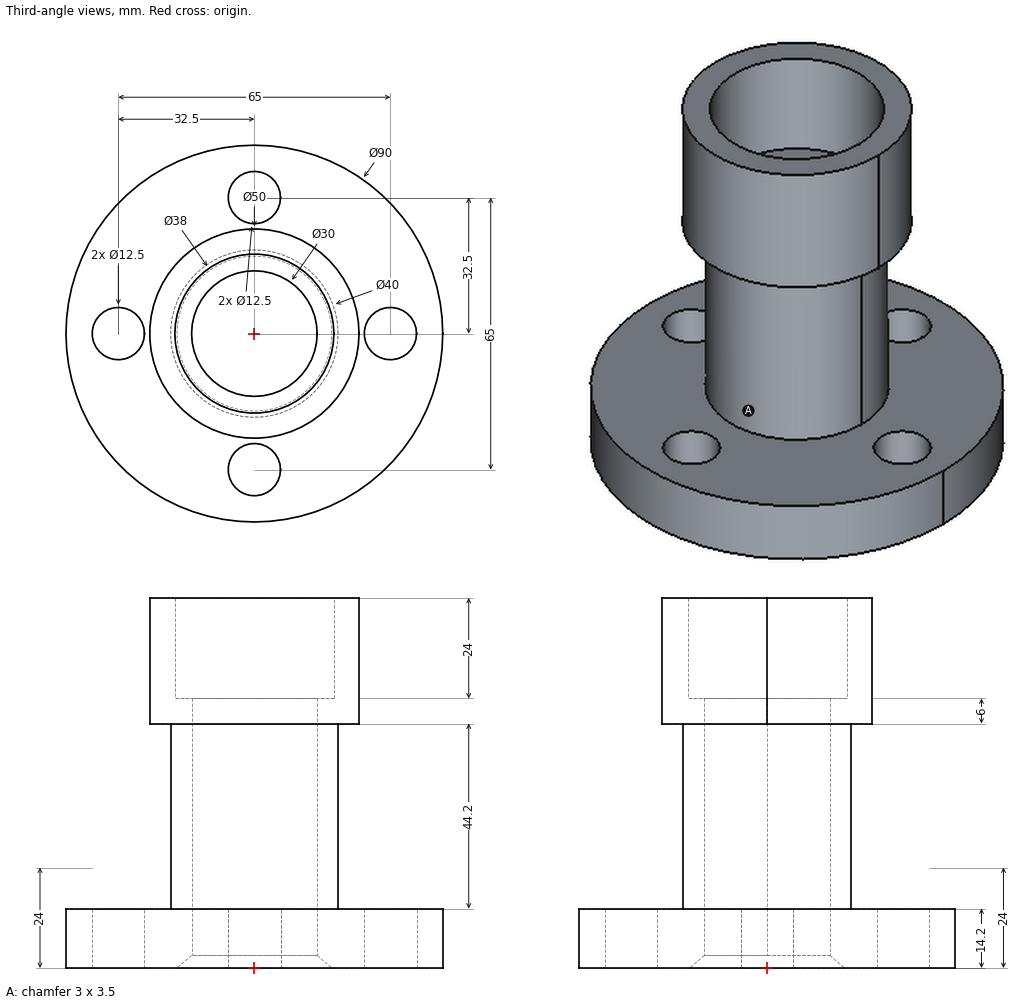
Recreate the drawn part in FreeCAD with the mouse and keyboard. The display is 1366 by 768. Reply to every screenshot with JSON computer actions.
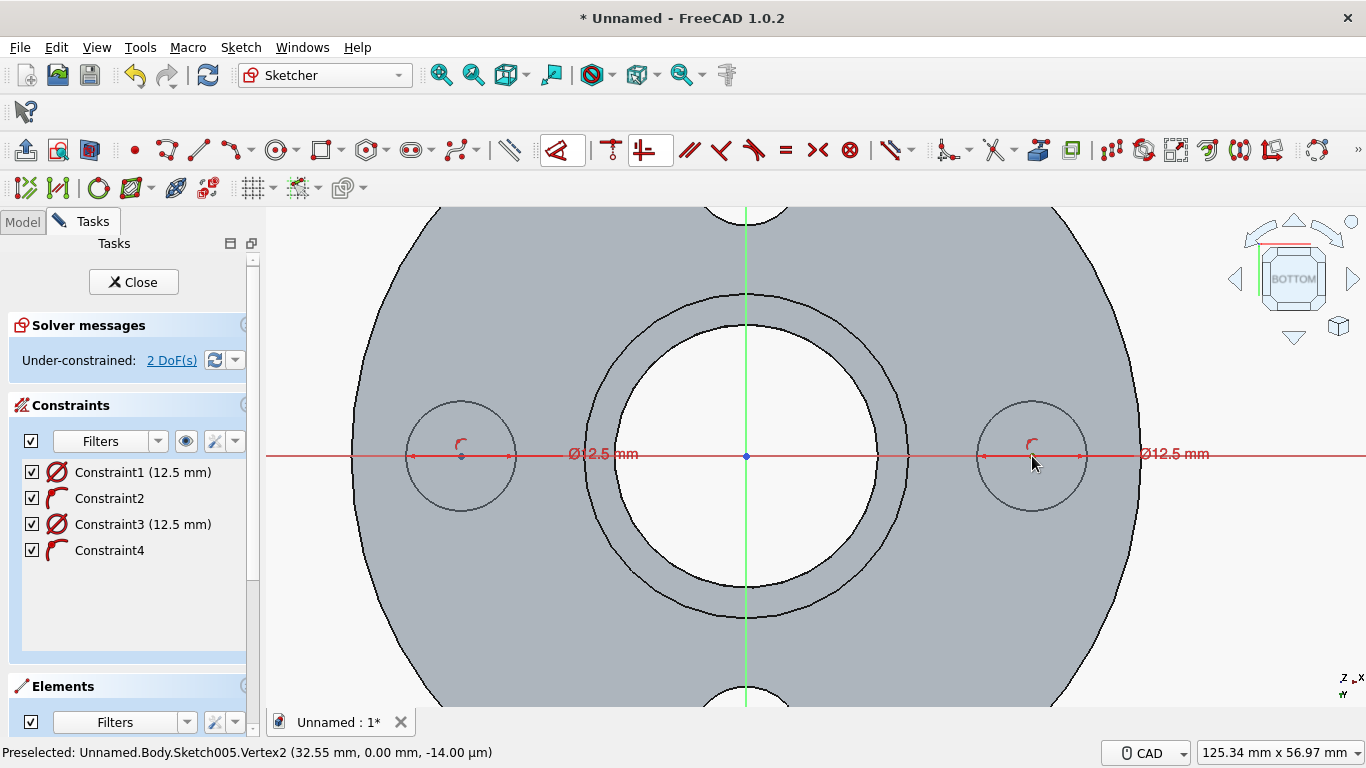
{"action": "left_click", "coordinate": [580, 150]}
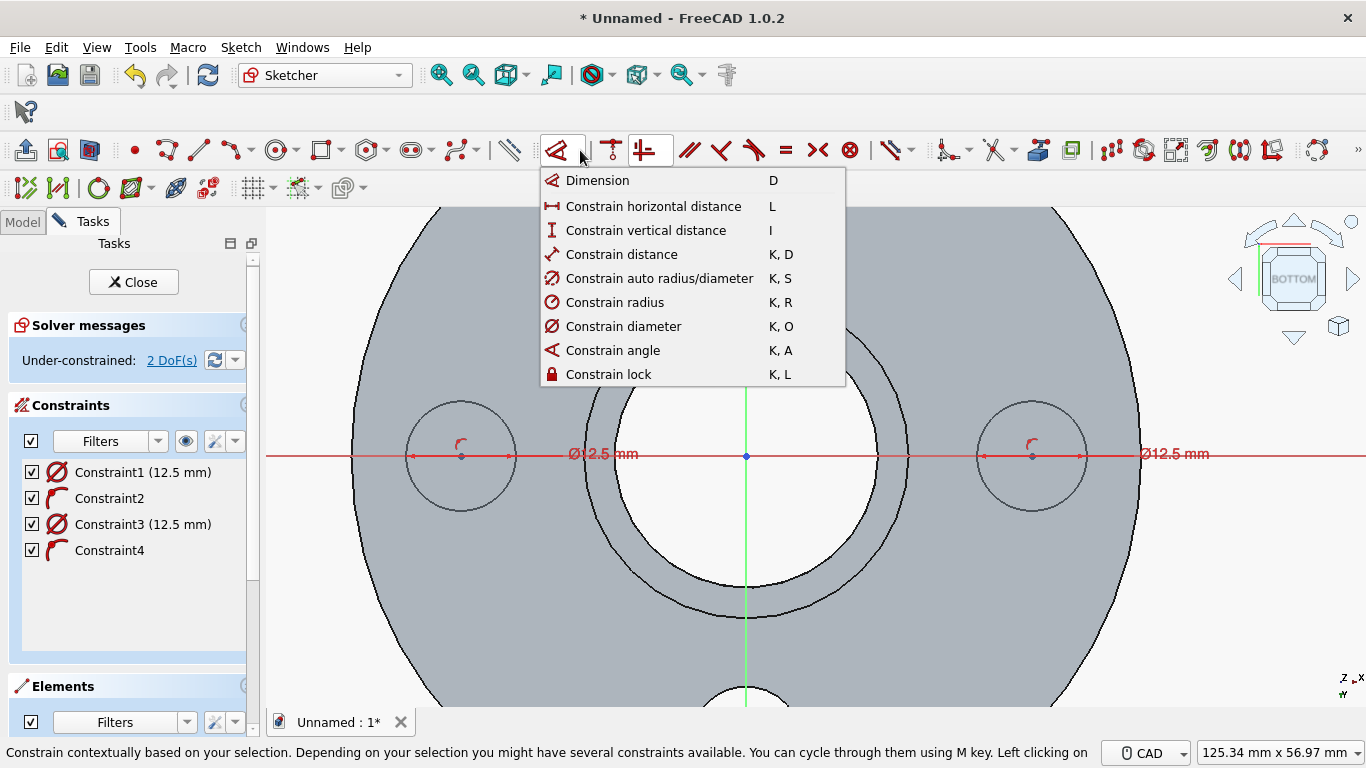
{"action": "left_click", "coordinate": [693, 206]}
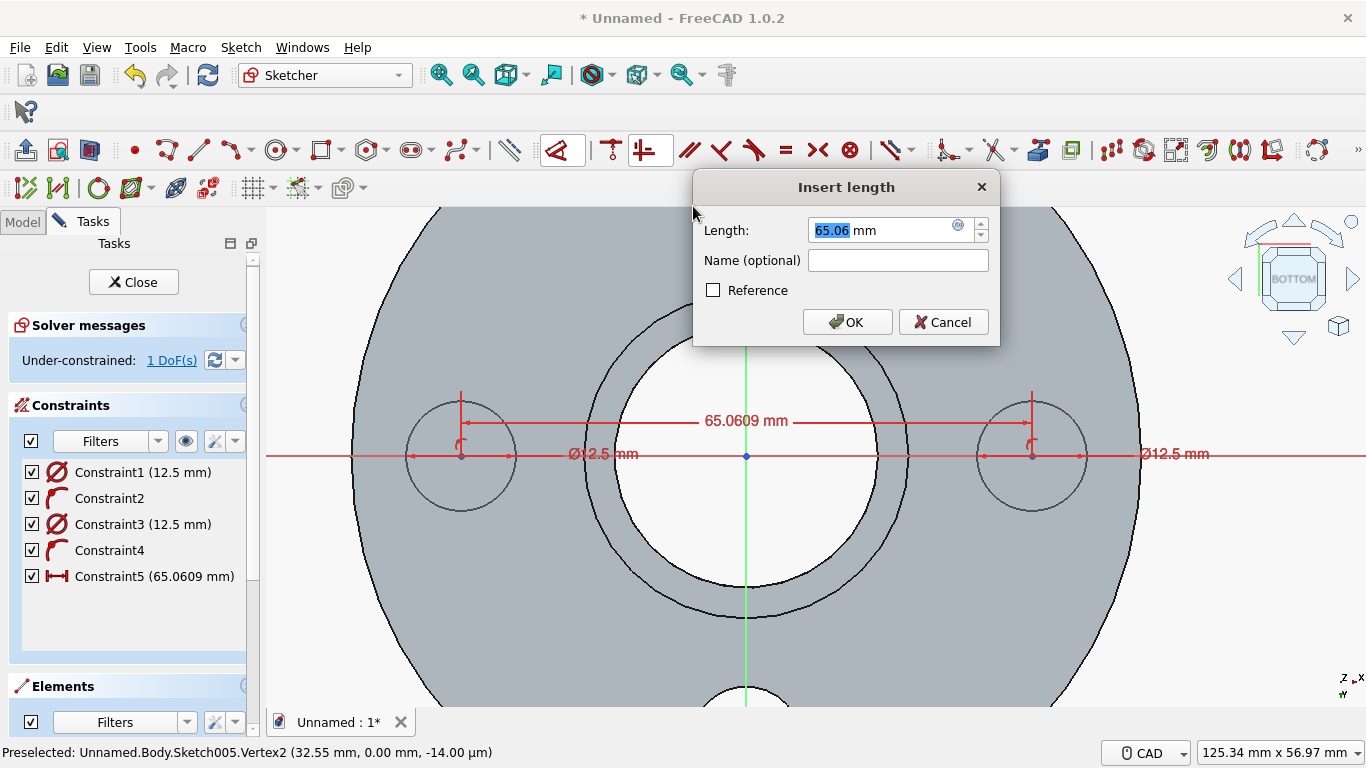
{"action": "type", "text": "65"}
{"action": "key", "text": "Return"}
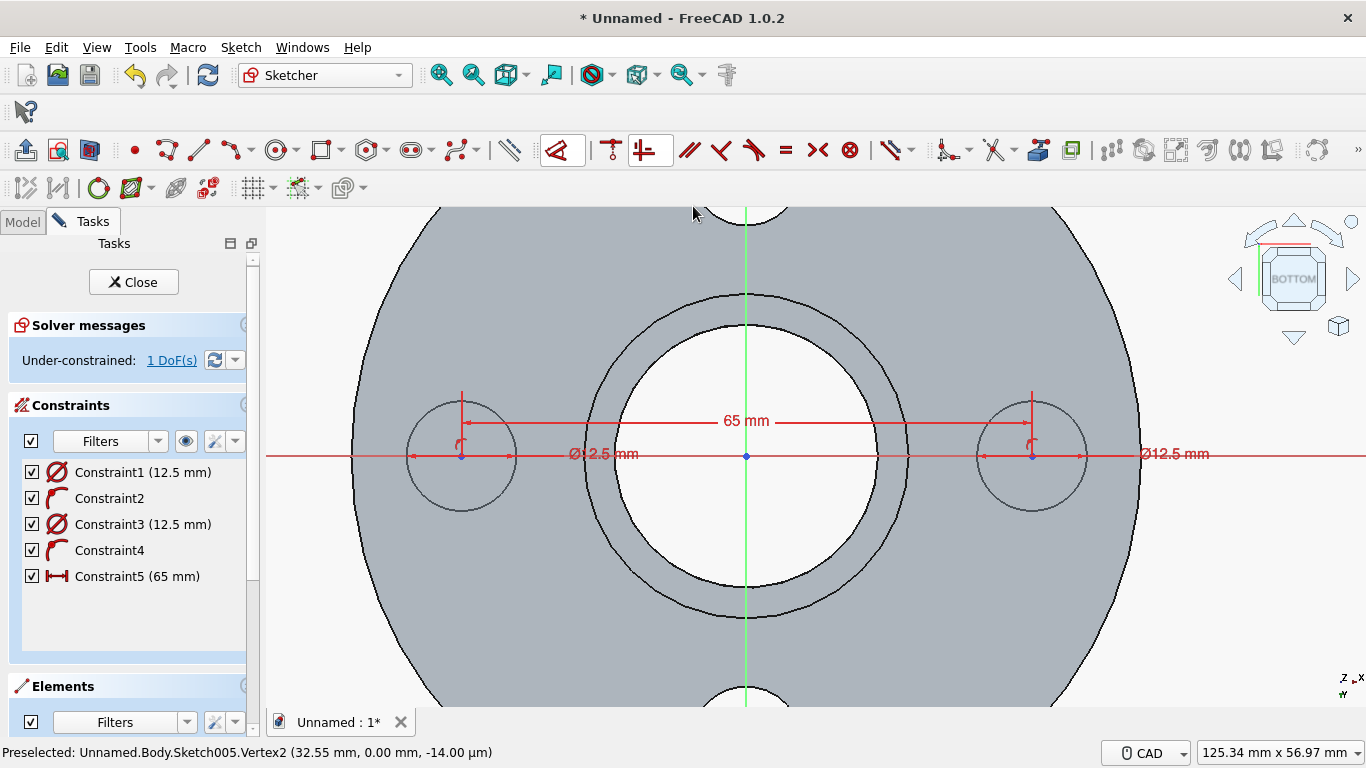
{"action": "left_click", "coordinate": [462, 456]}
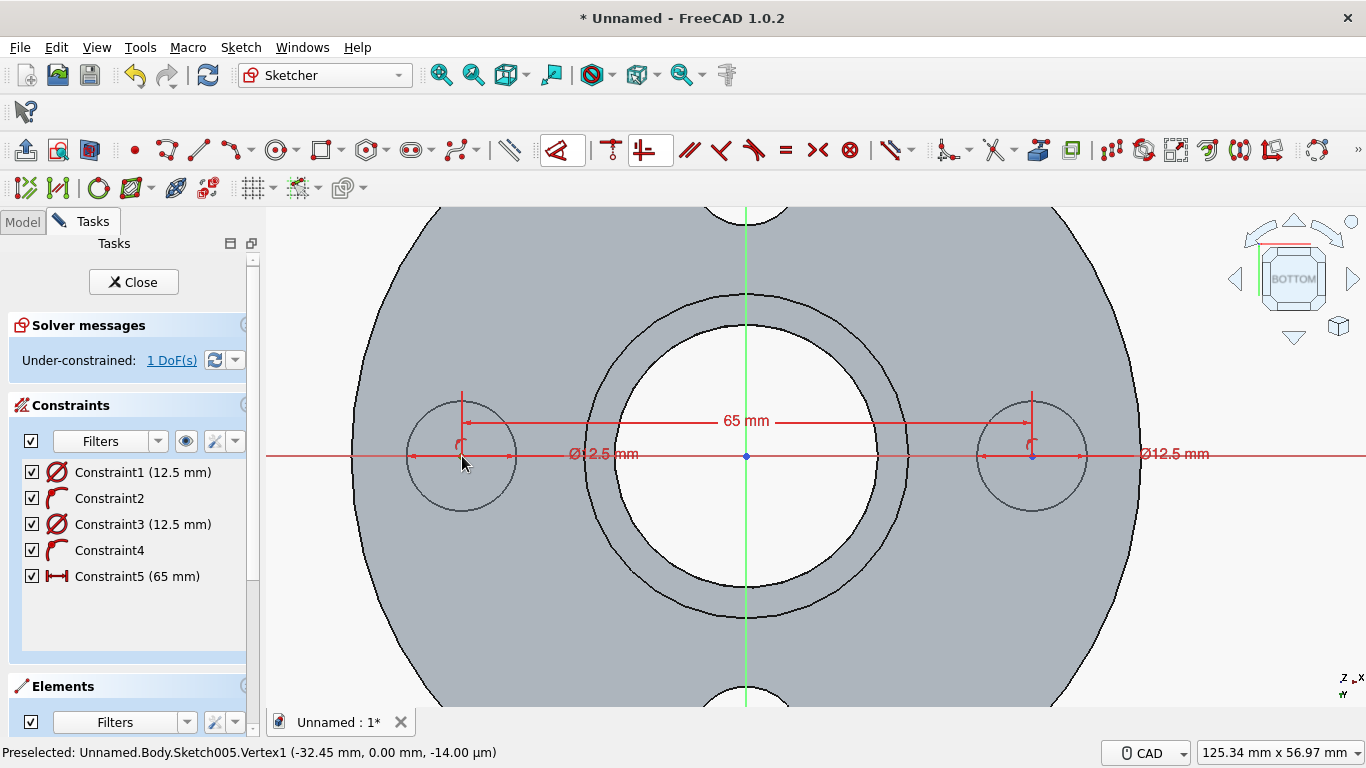
{"action": "left_click", "coordinate": [580, 150]}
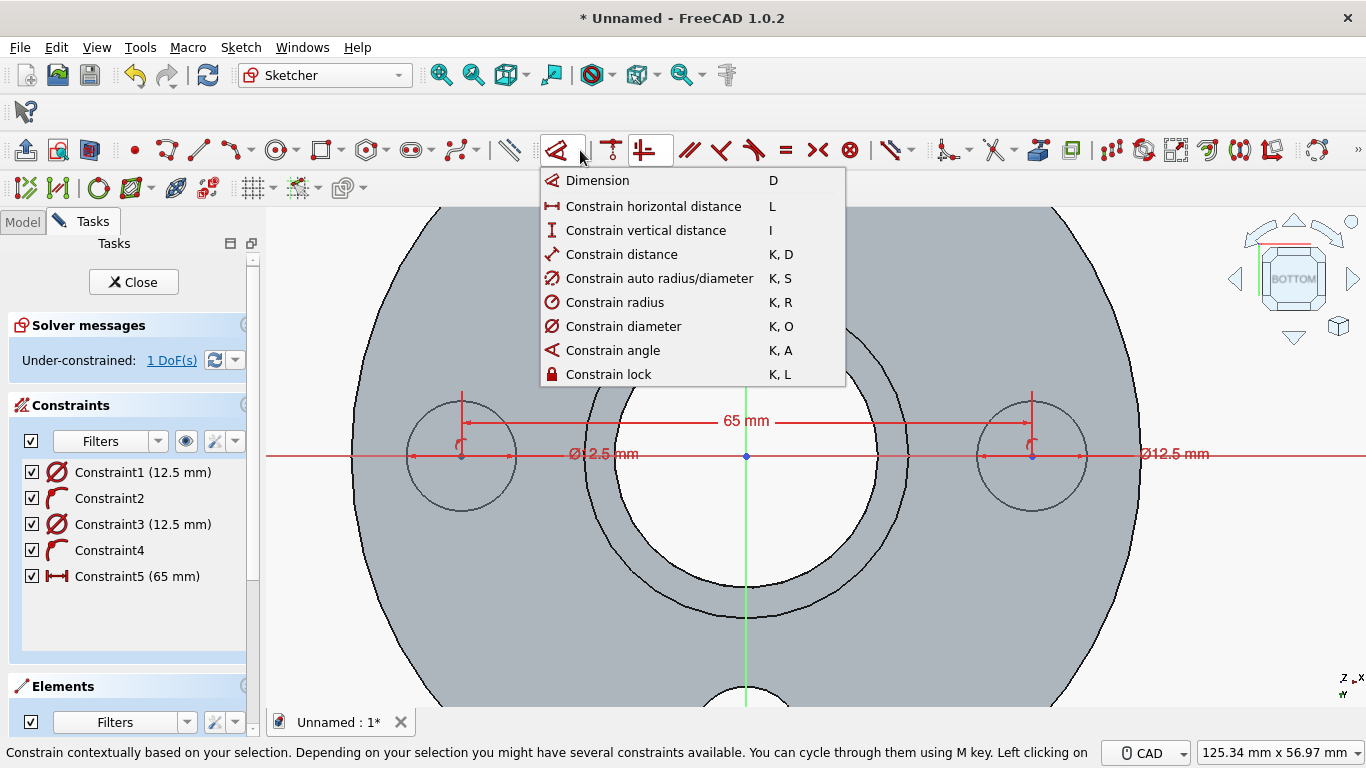
{"action": "left_click", "coordinate": [693, 206]}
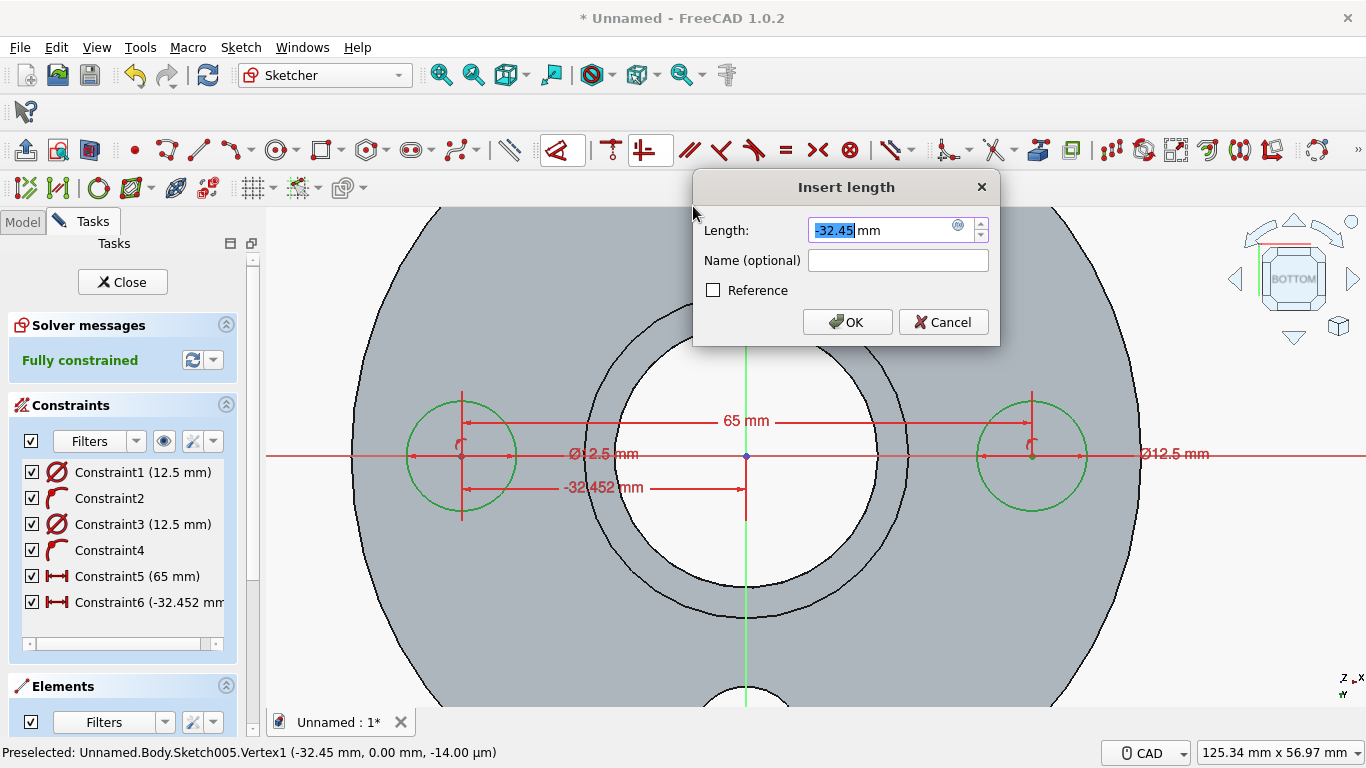
{"action": "type", "text": "-32.5"}
{"action": "key", "text": "Return"}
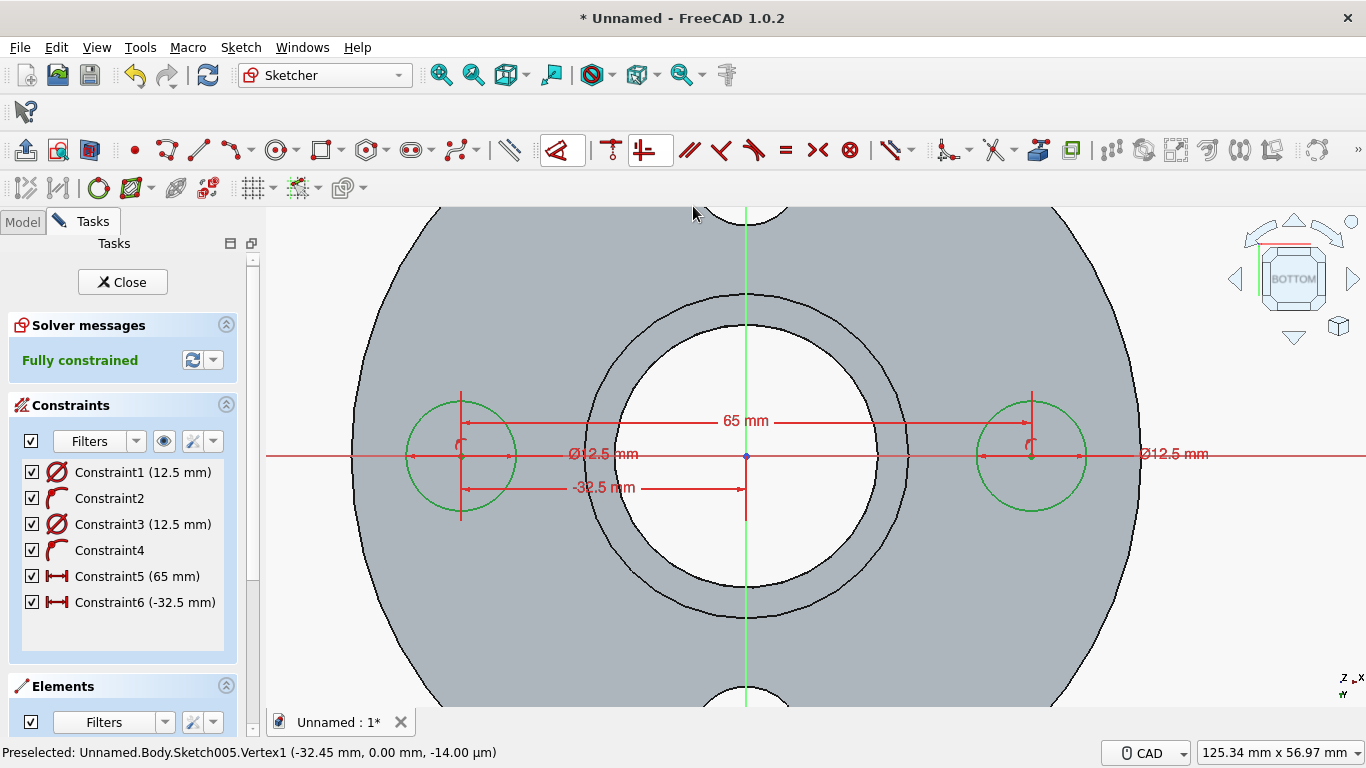
{"action": "left_click", "coordinate": [123, 282]}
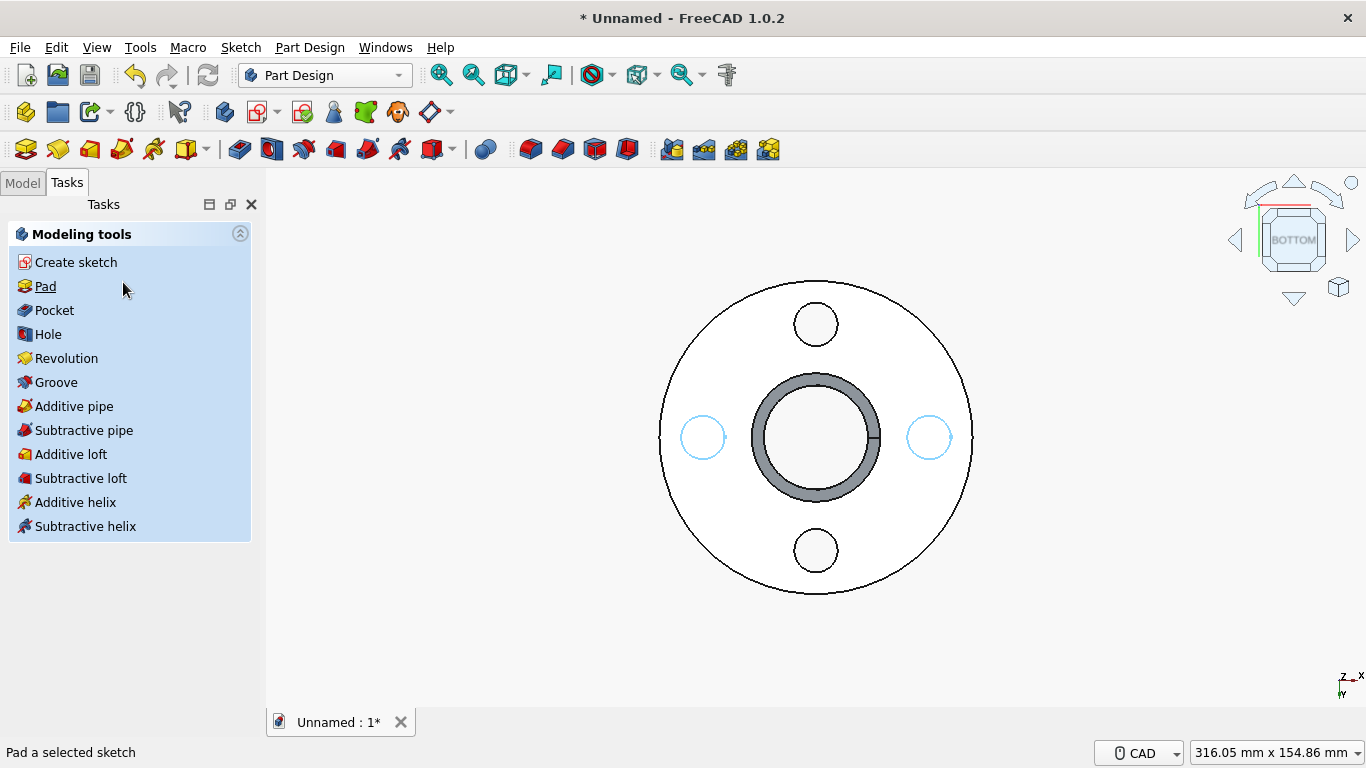
{"action": "left_click", "coordinate": [240, 150]}